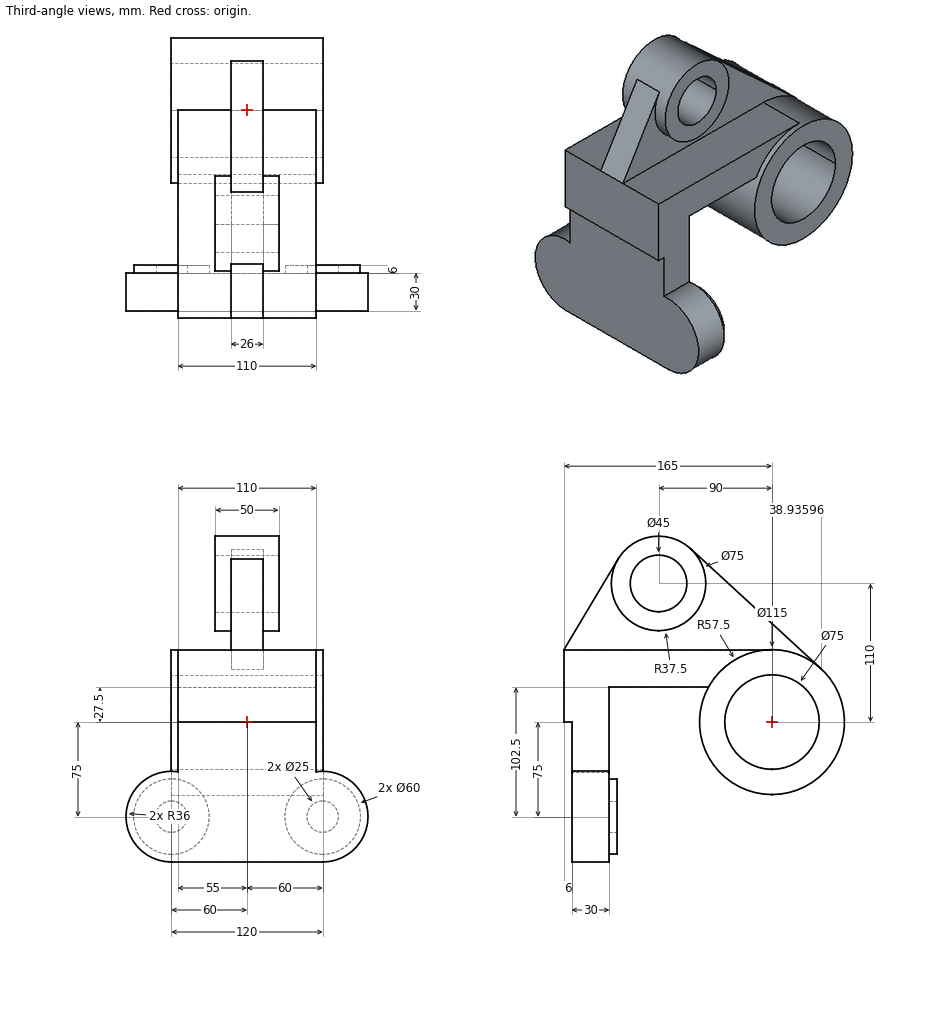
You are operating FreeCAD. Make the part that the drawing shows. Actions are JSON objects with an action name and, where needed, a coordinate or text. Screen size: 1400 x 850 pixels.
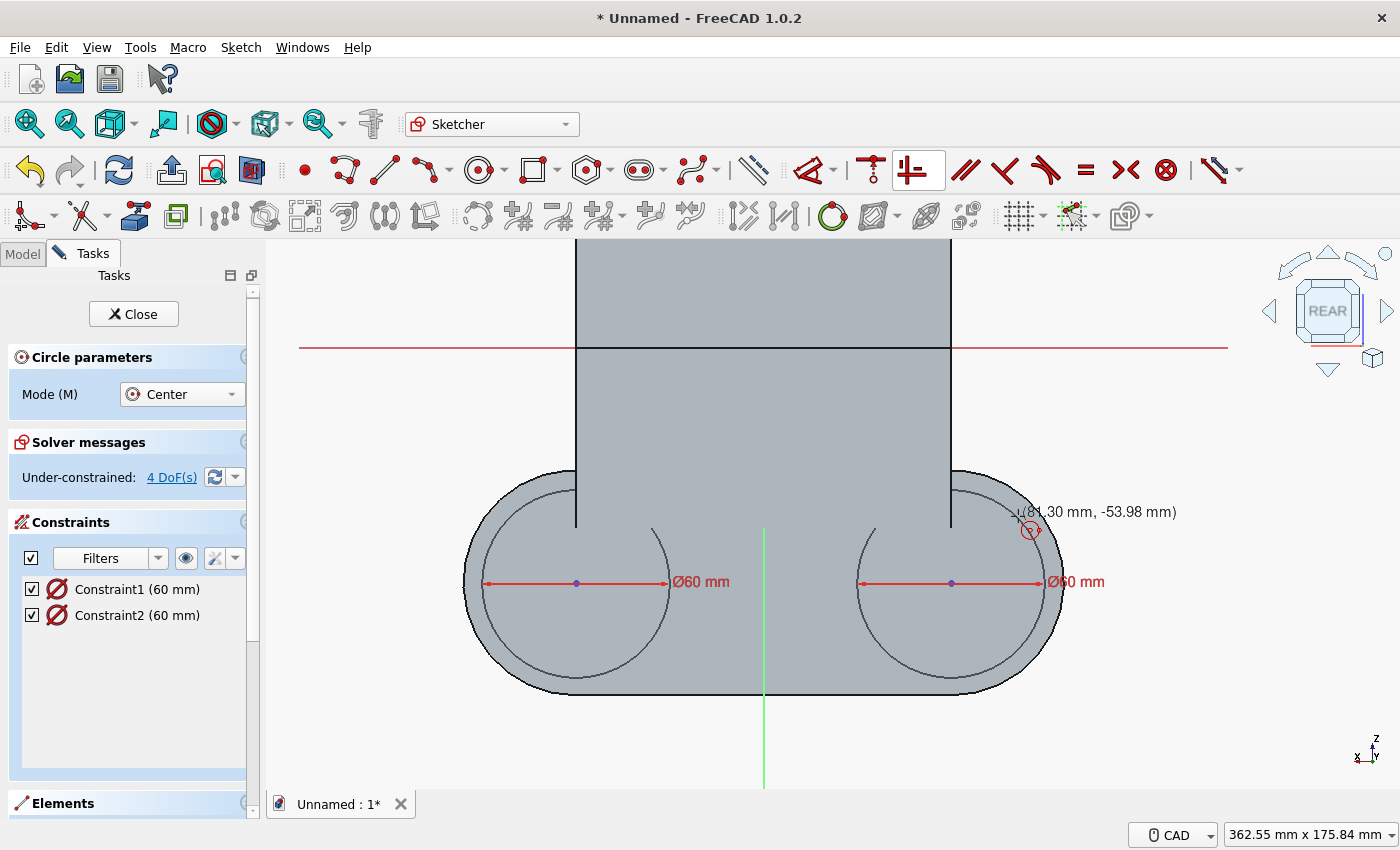
{"action": "left_click", "coordinate": [576, 584]}
{"action": "mouse_move", "coordinate": [604, 555]}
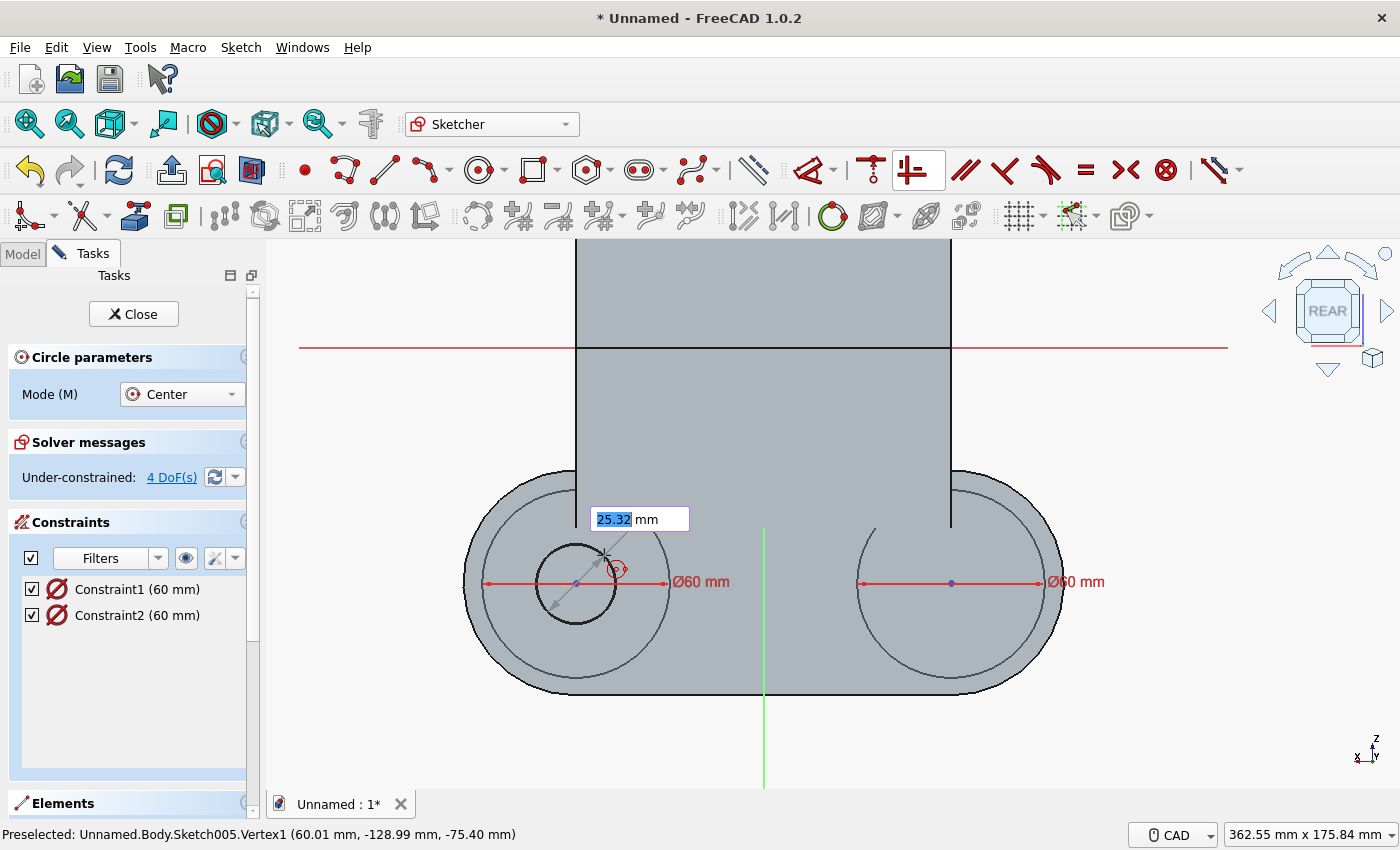
{"action": "type", "text": "25"}
{"action": "key", "text": "Return"}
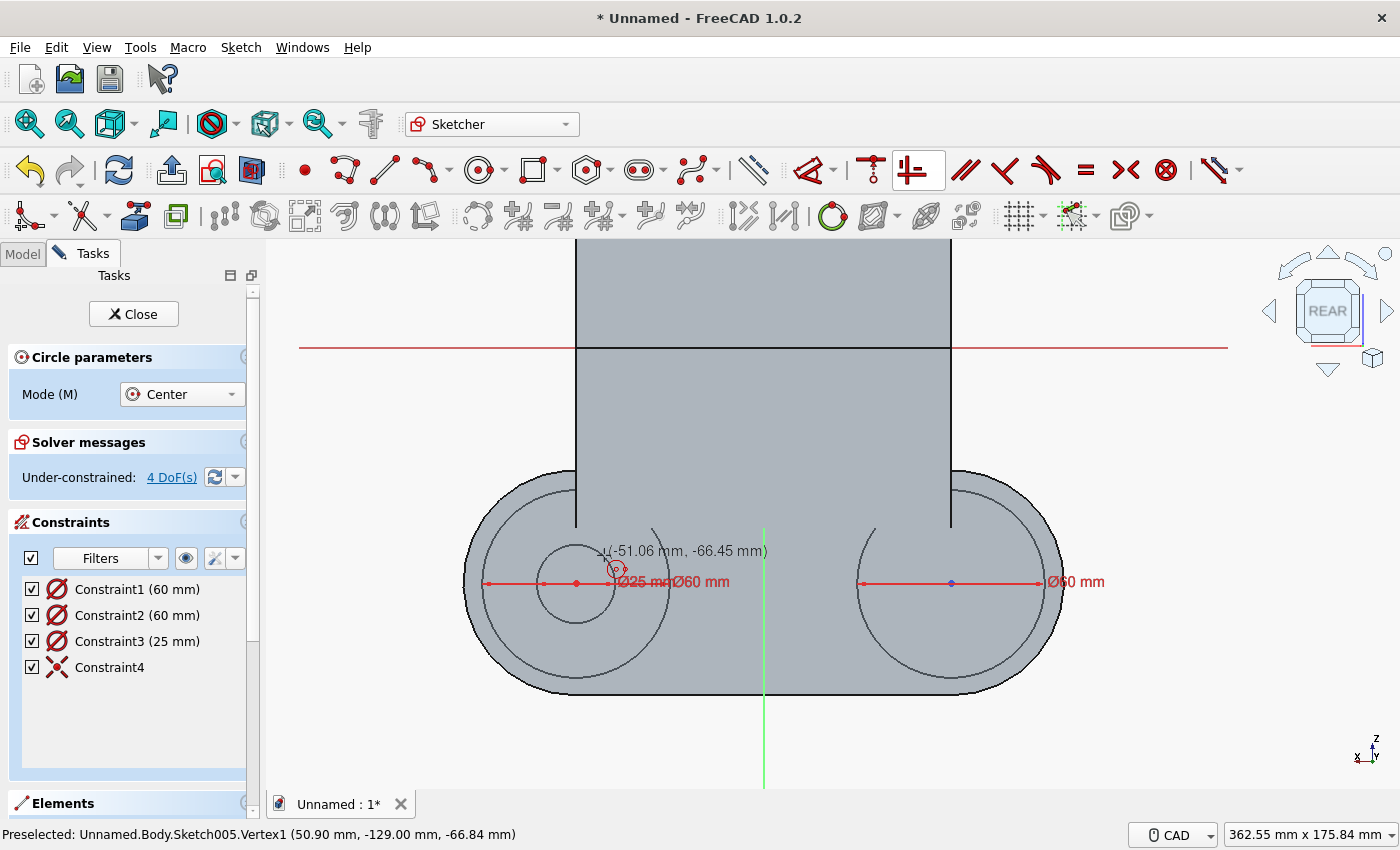
{"action": "left_click", "coordinate": [951, 584]}
{"action": "mouse_move", "coordinate": [979, 555]}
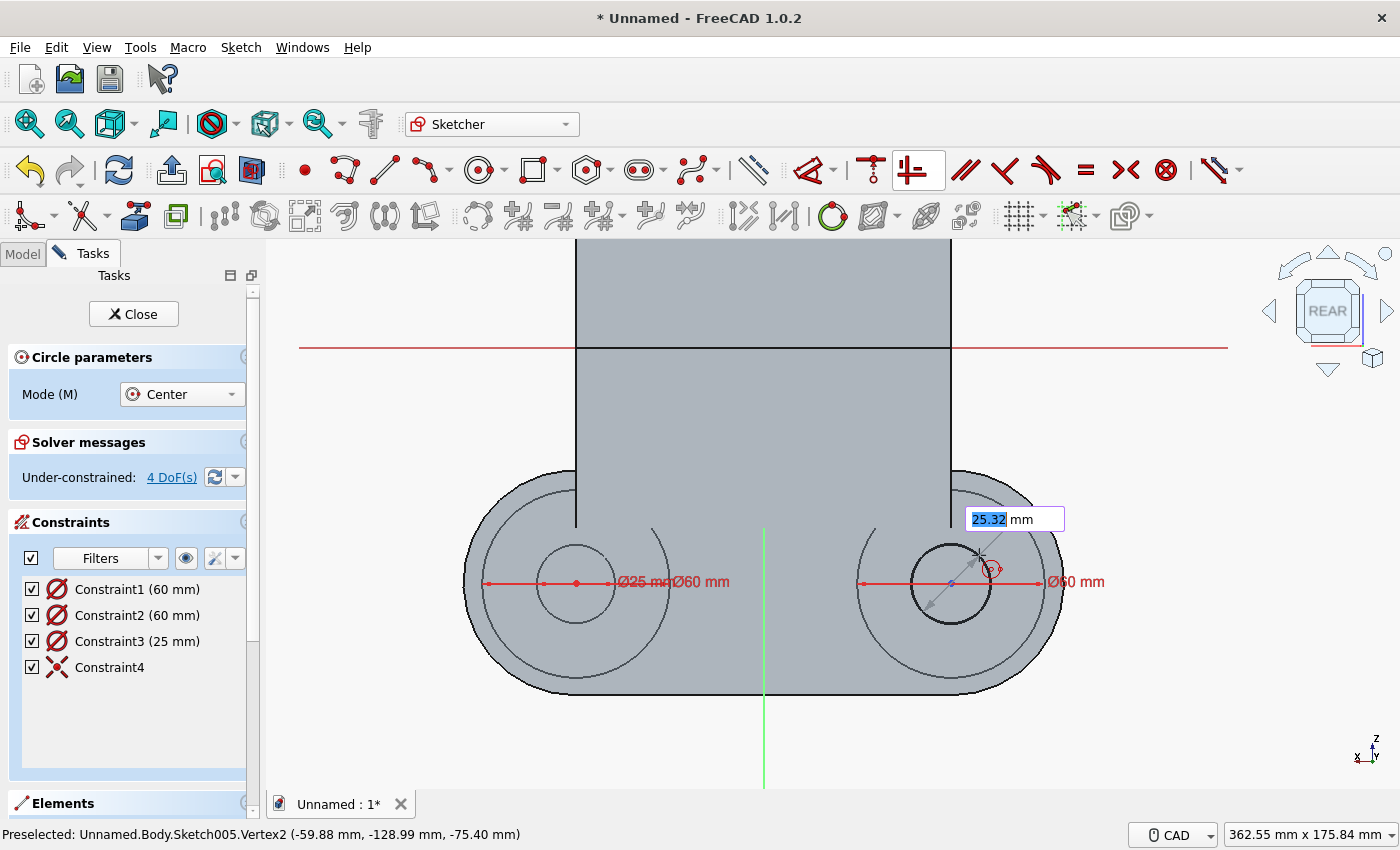
{"action": "type", "text": "25"}
{"action": "key", "text": "Return"}
{"action": "key", "text": "Escape"}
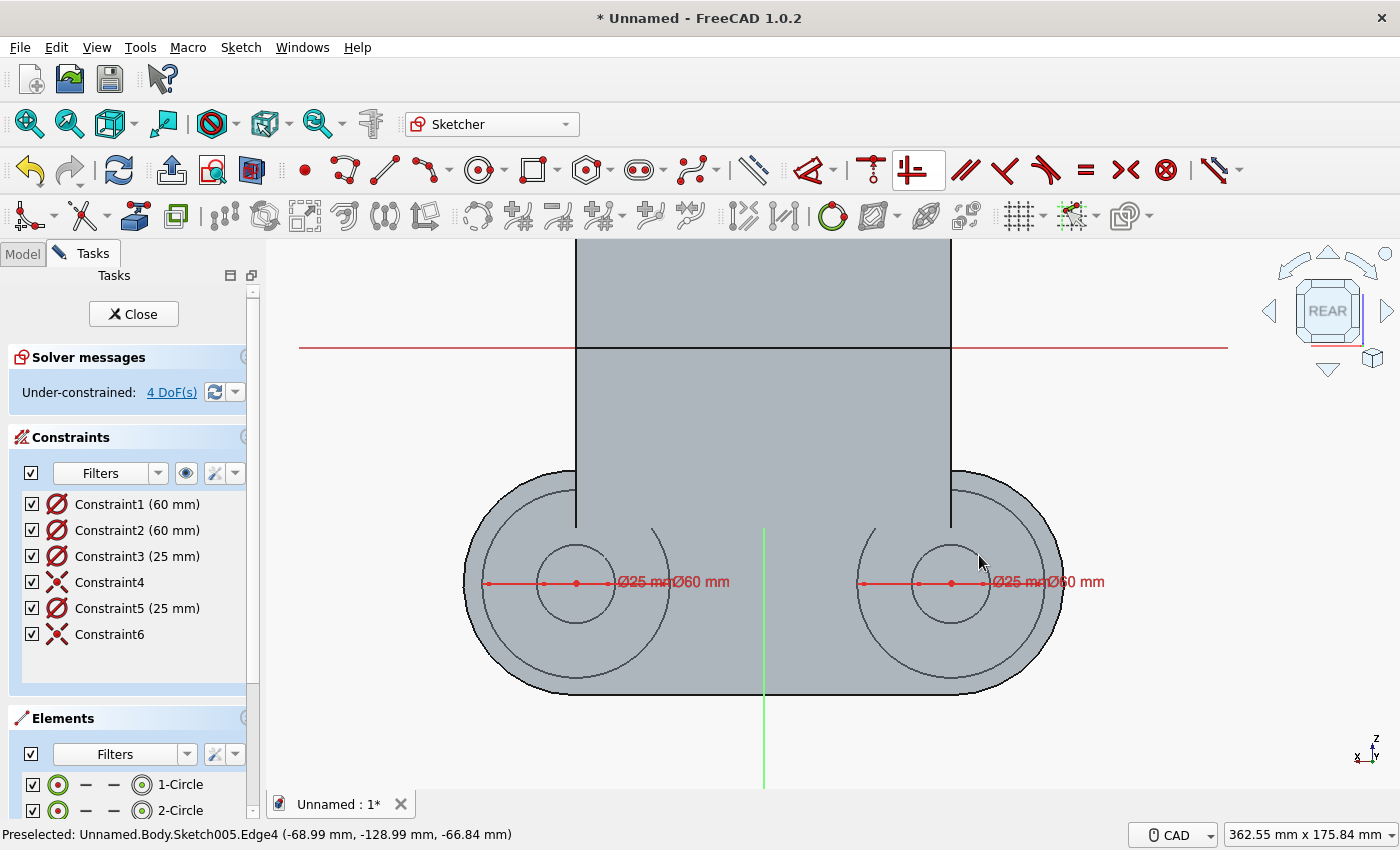
{"action": "key", "text": "d"}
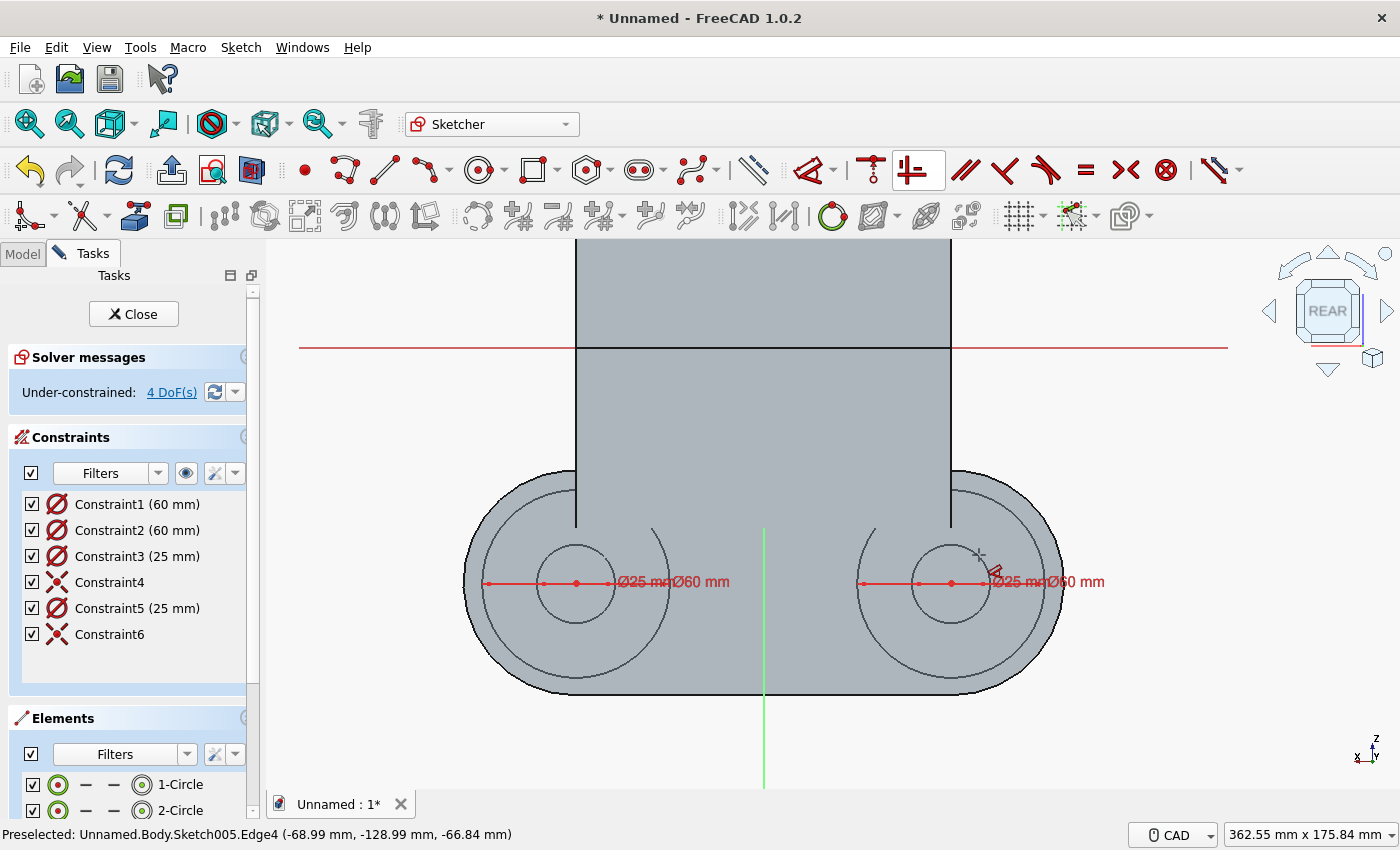
{"action": "left_click", "coordinate": [576, 584]}
{"action": "left_click", "coordinate": [670, 314]}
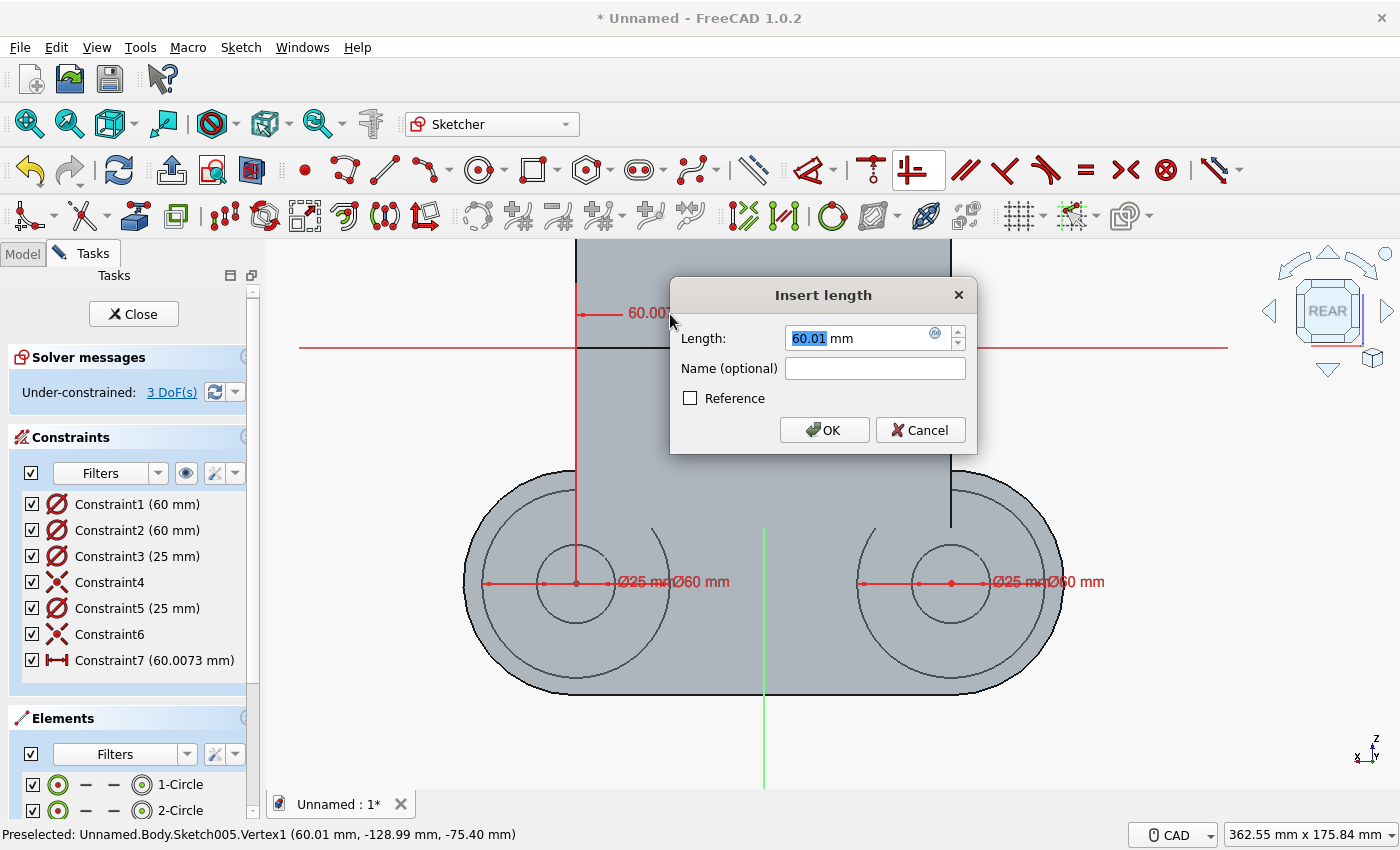
{"action": "type", "text": "60"}
{"action": "key", "text": "Return"}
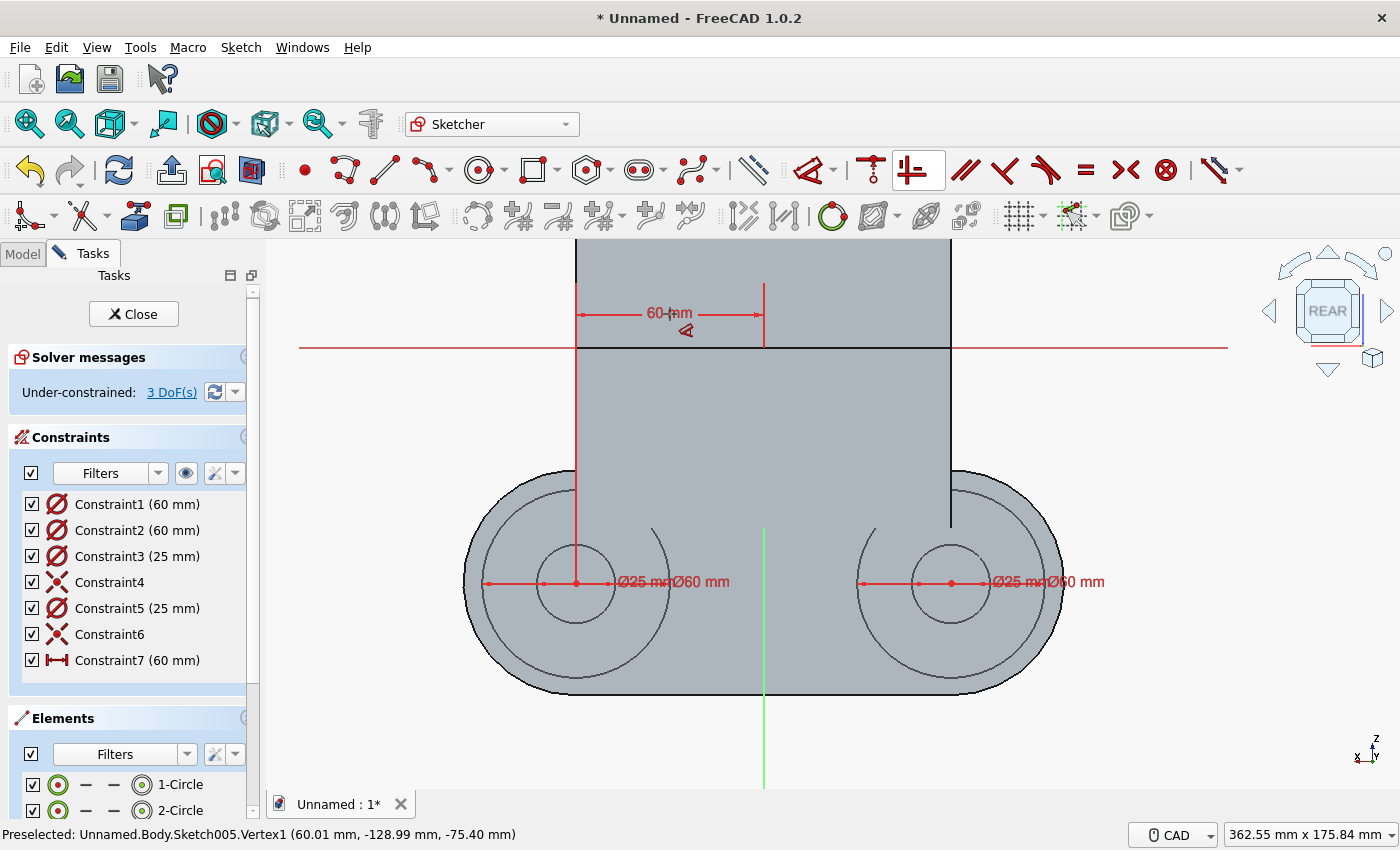
{"action": "left_click", "coordinate": [576, 584]}
{"action": "left_click", "coordinate": [542, 466]}